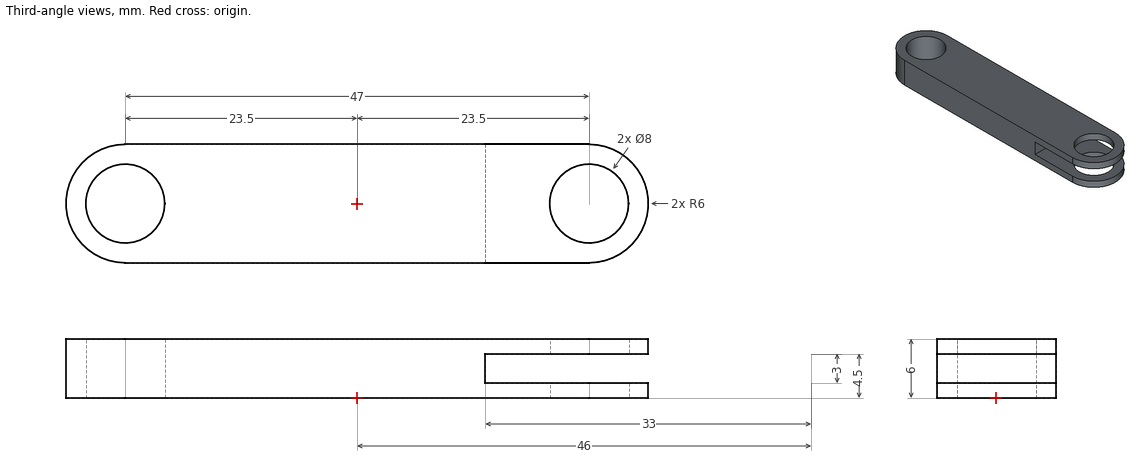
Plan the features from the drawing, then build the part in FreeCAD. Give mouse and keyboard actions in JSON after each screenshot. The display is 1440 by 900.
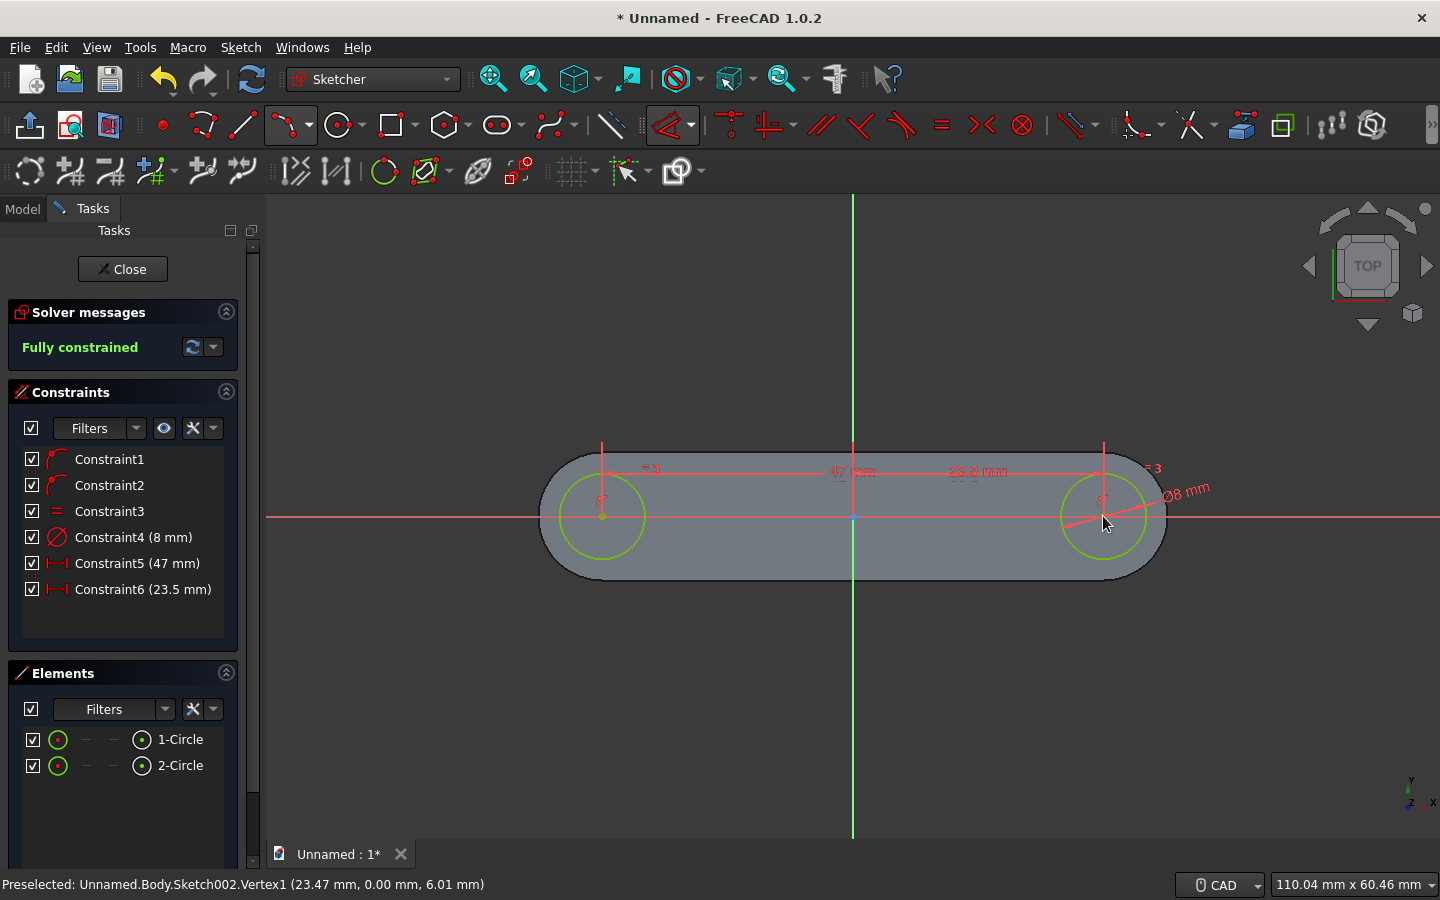
{"action": "left_click", "coordinate": [123, 269]}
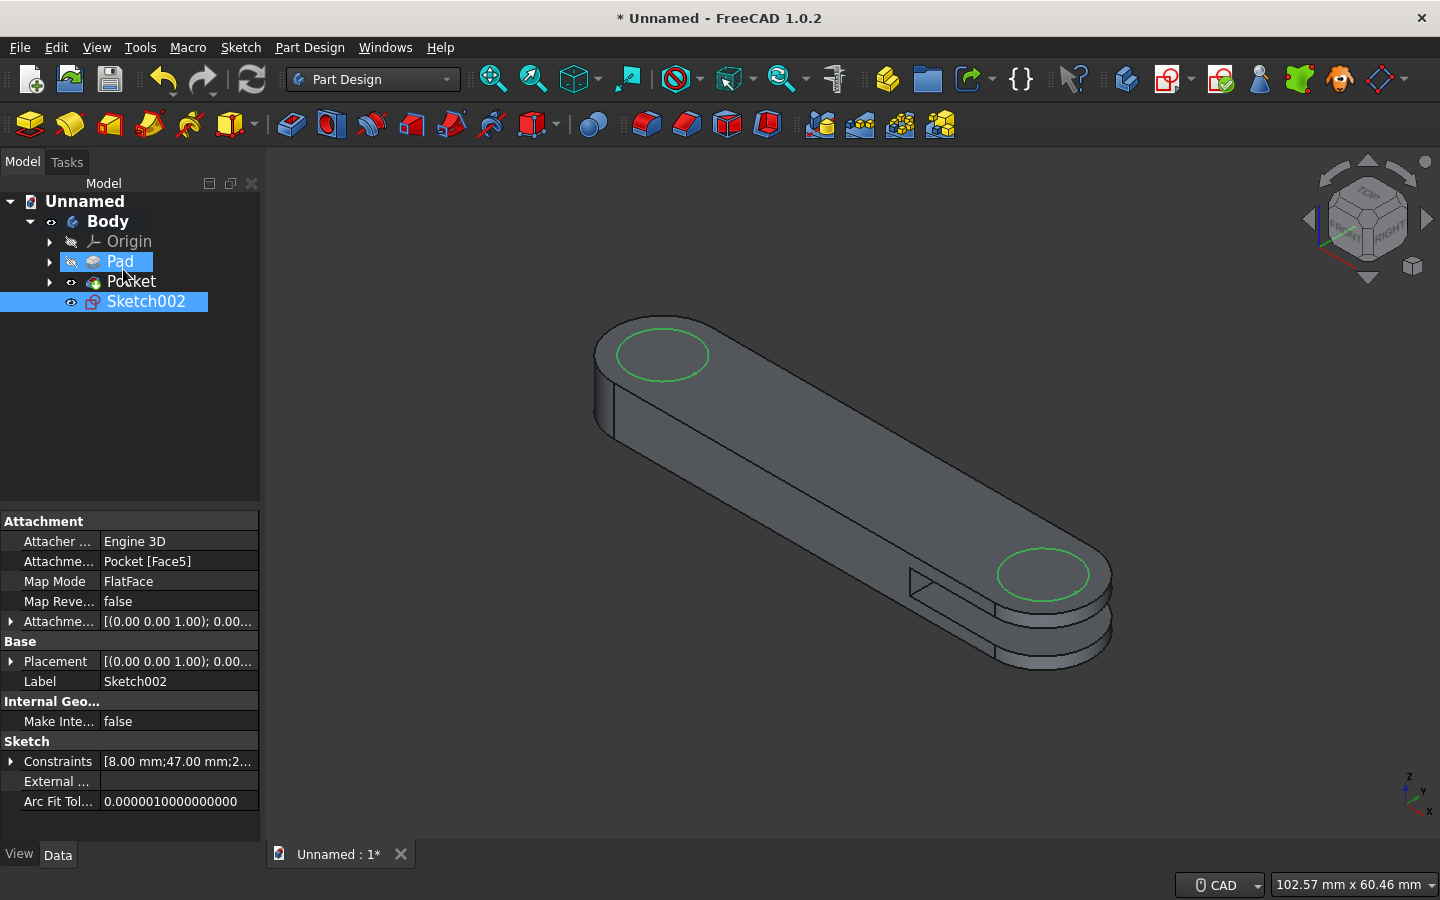
{"action": "left_click", "coordinate": [292, 124]}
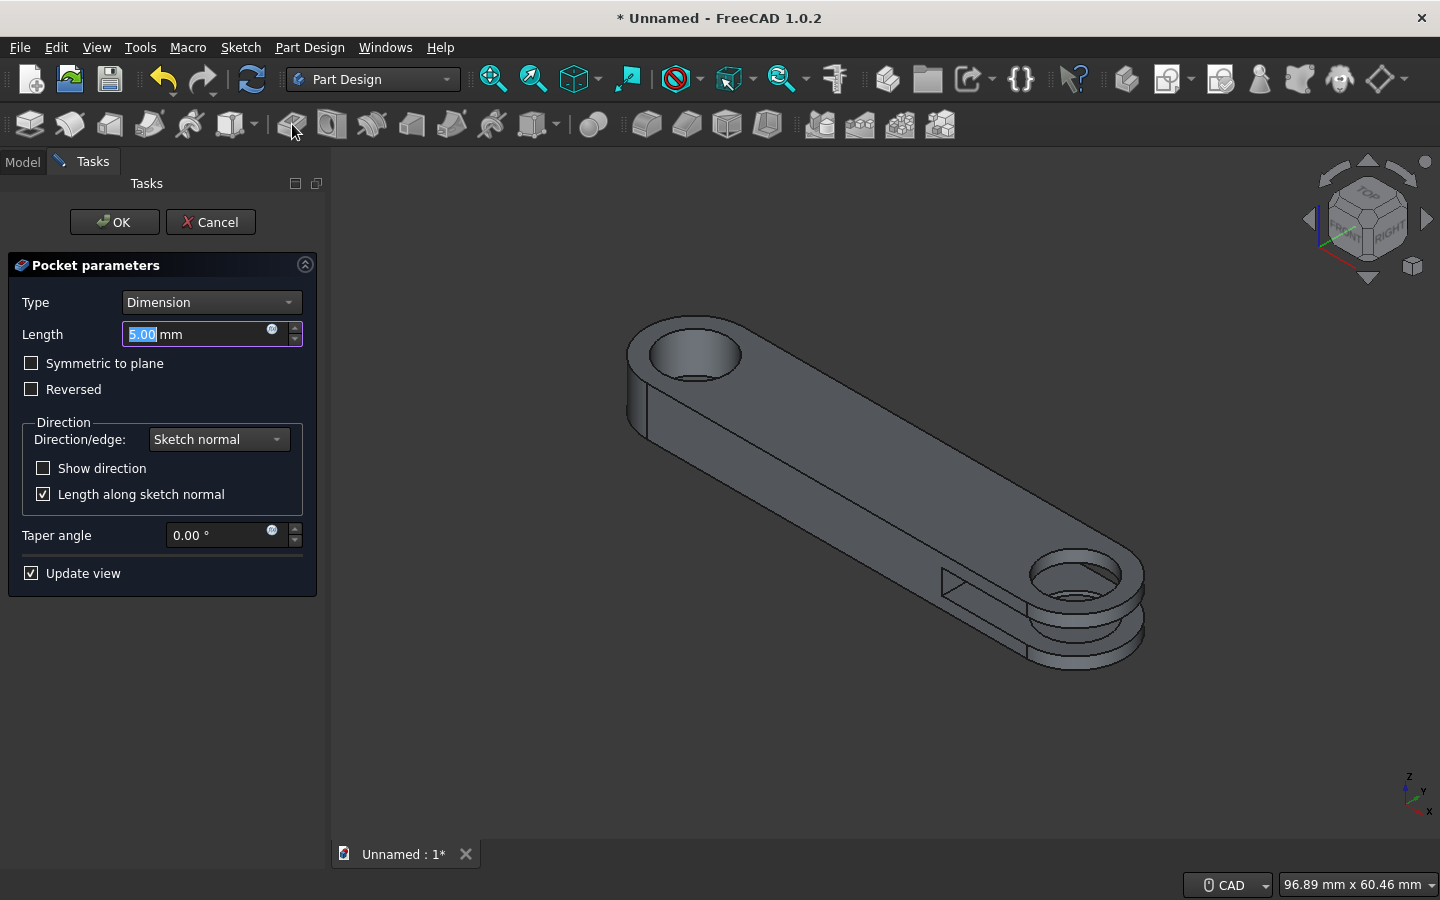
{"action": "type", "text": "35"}
{"action": "key", "text": "Tab"}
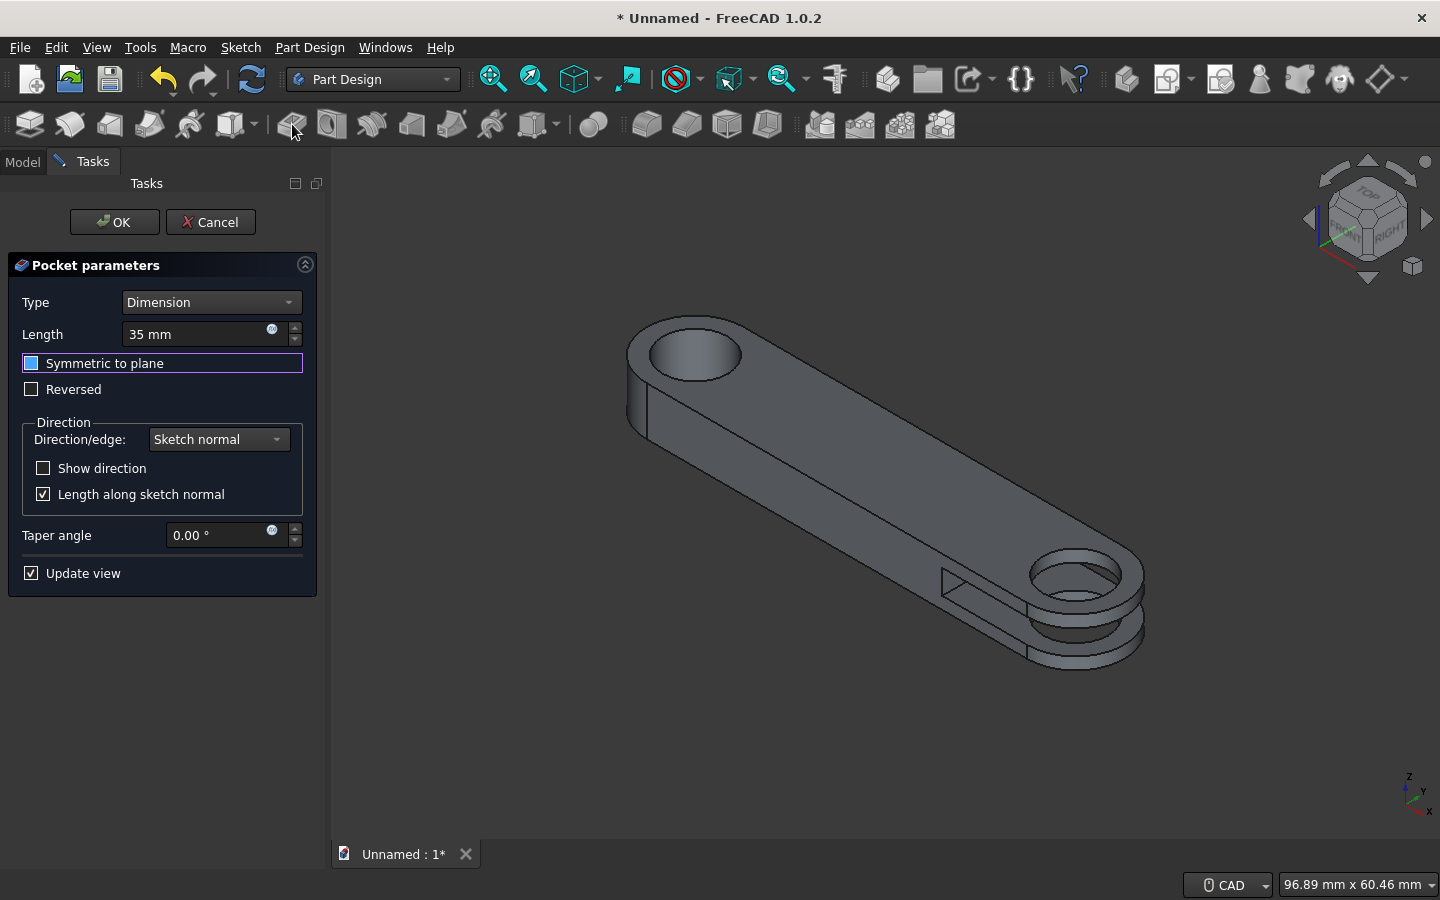
{"action": "left_click", "coordinate": [115, 222]}